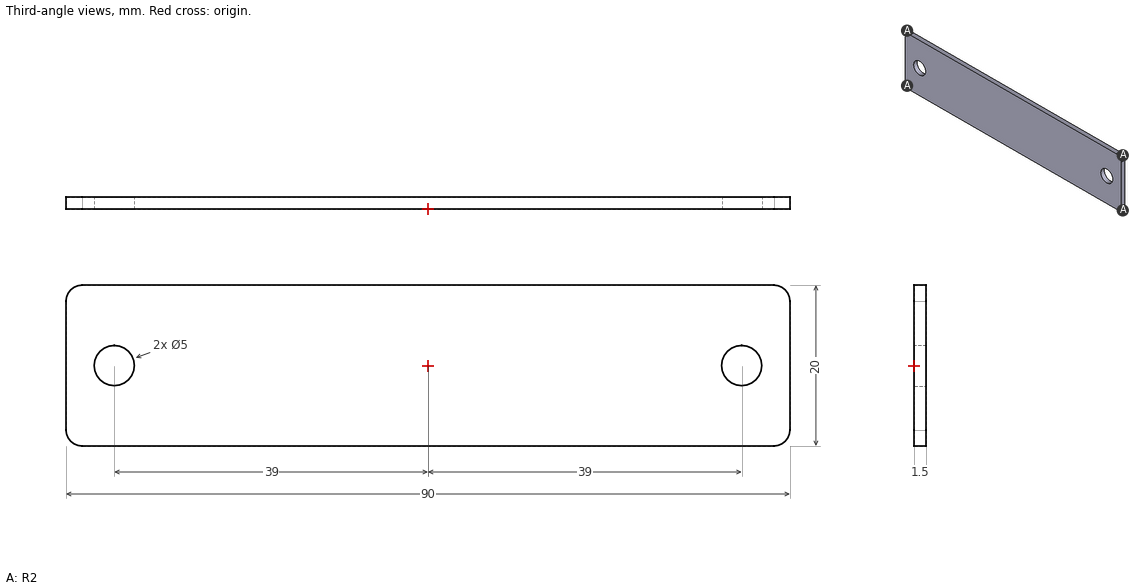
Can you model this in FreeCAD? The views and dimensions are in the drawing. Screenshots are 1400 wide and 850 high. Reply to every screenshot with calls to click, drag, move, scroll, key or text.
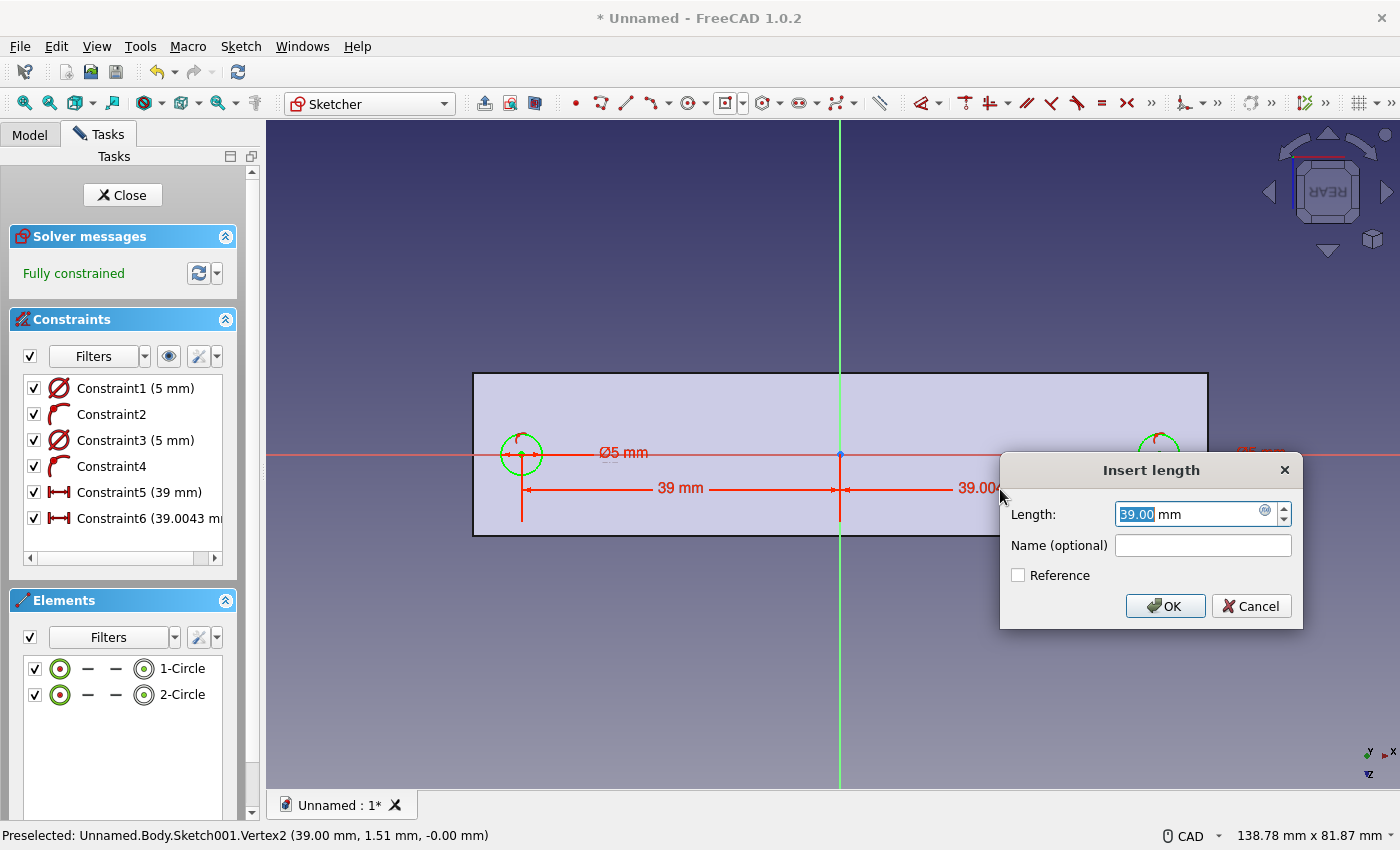
text(39)
key(Return)
key(Escape)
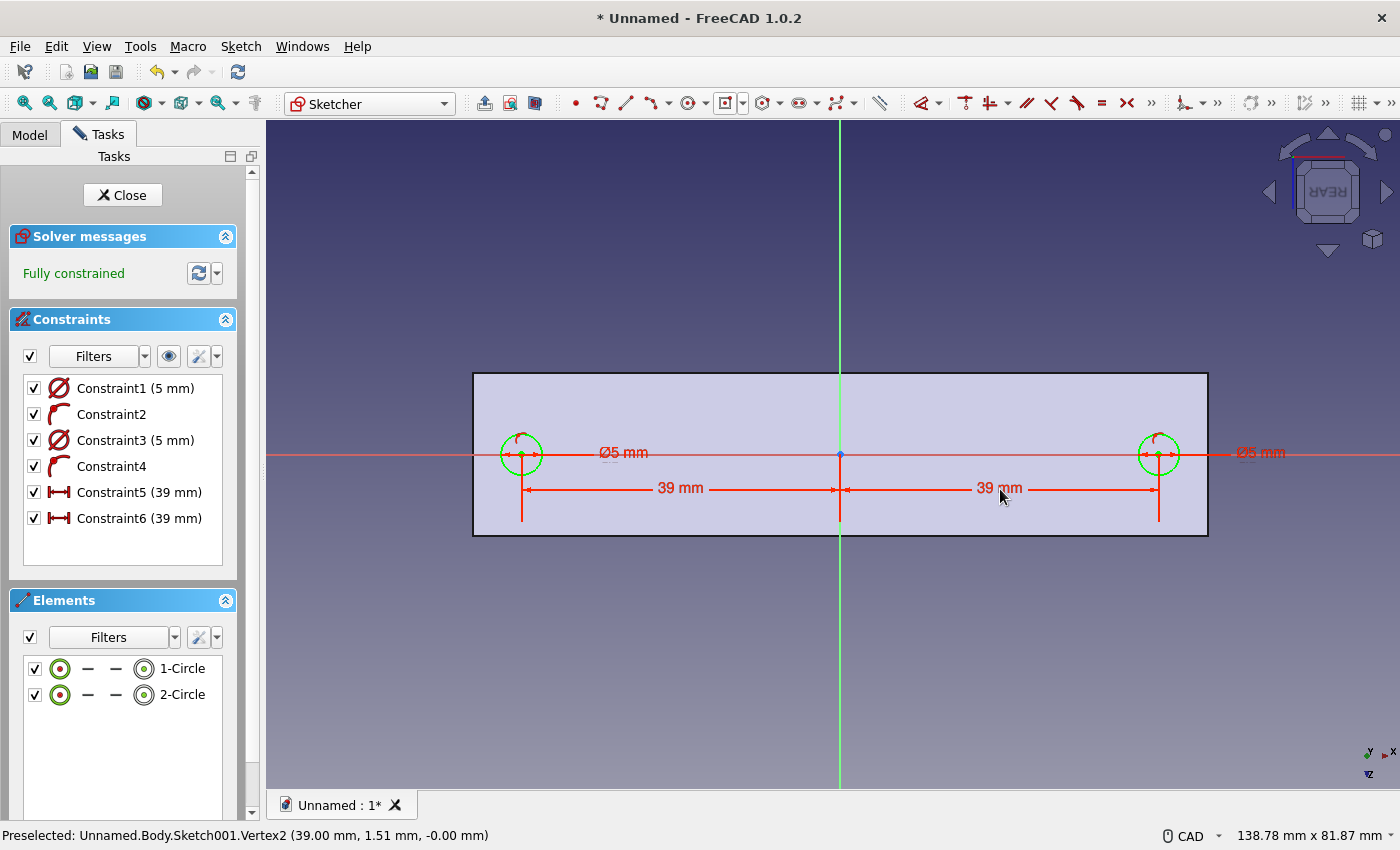
click(123, 195)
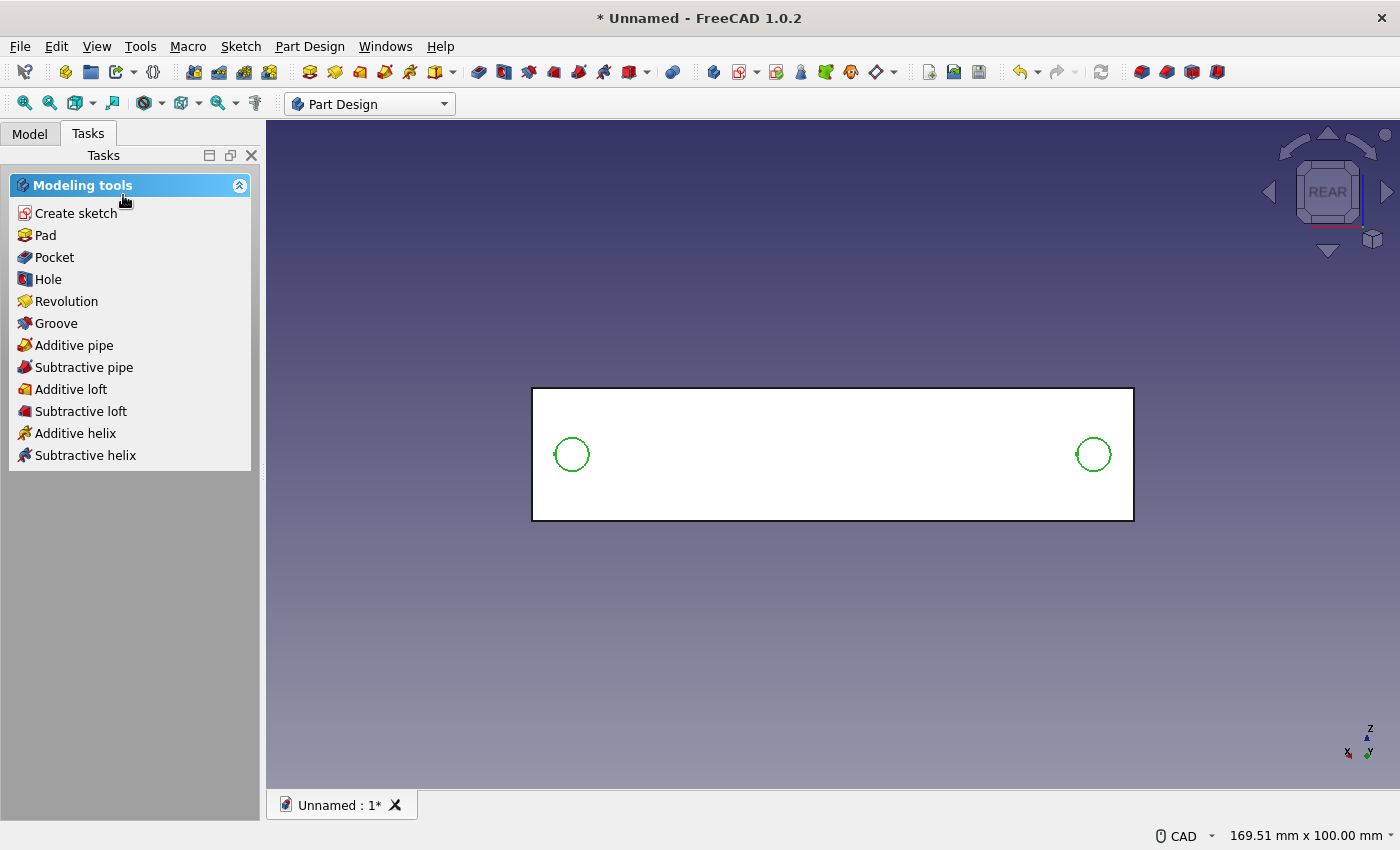
click(479, 72)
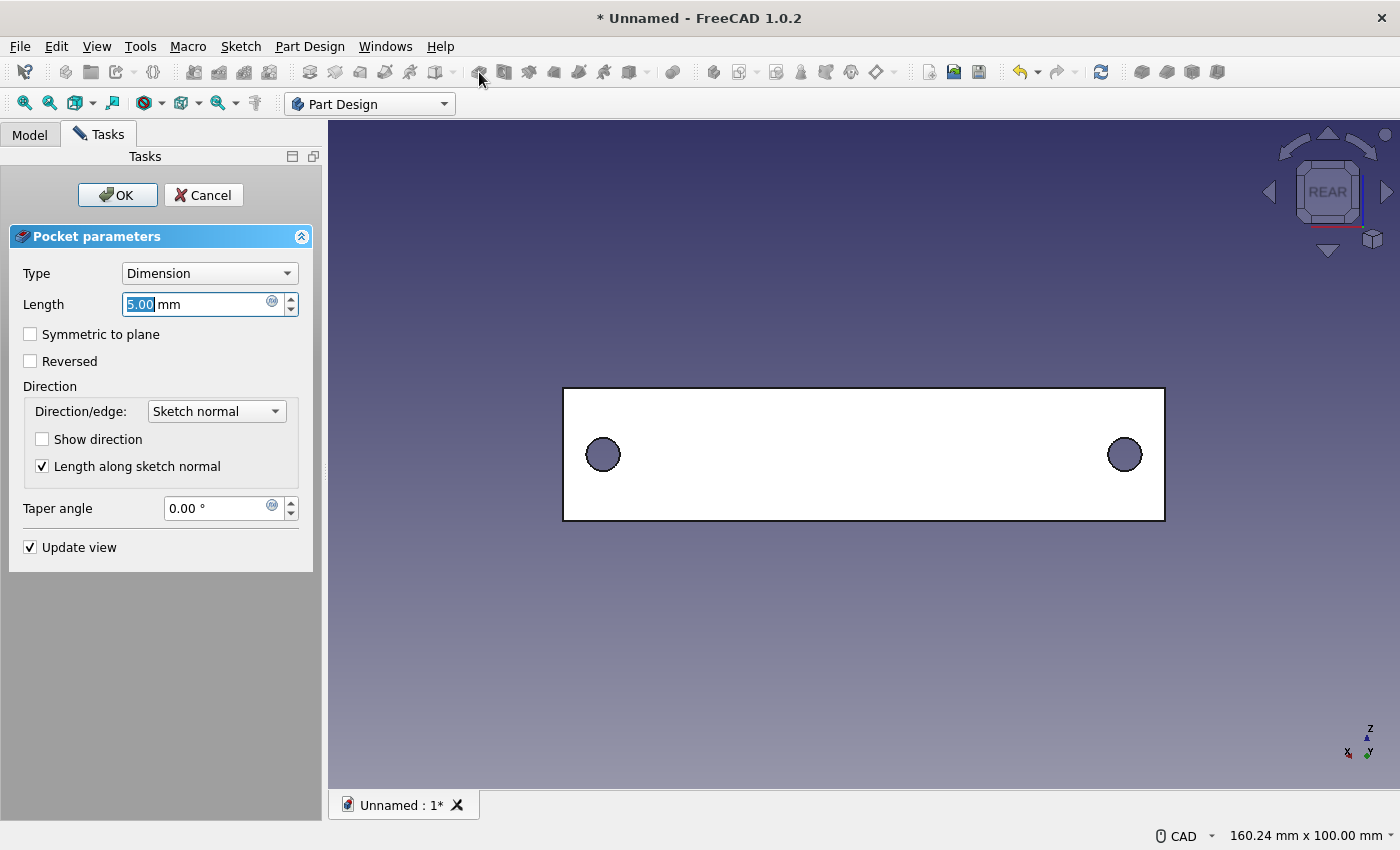
click(210, 274)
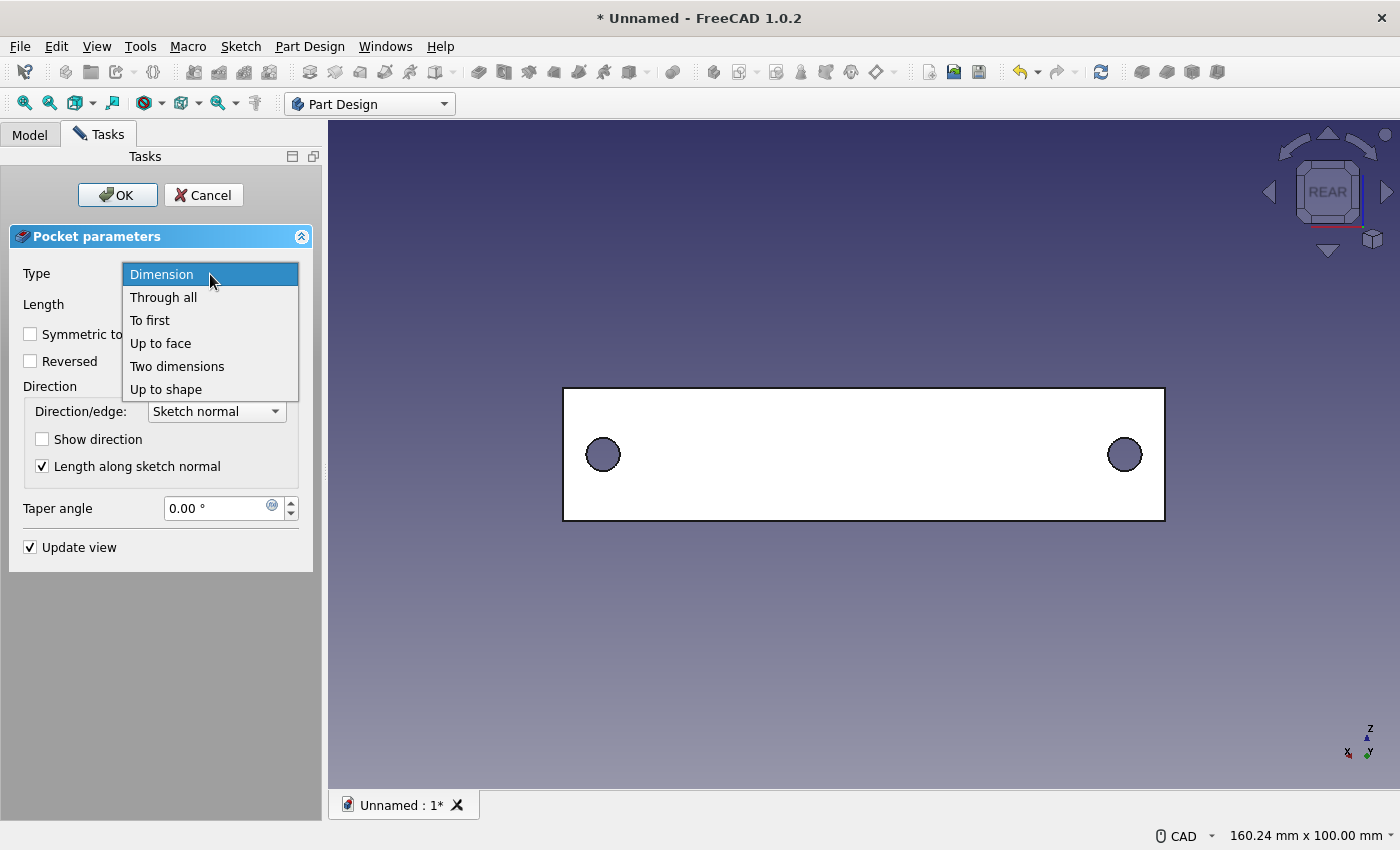
click(208, 298)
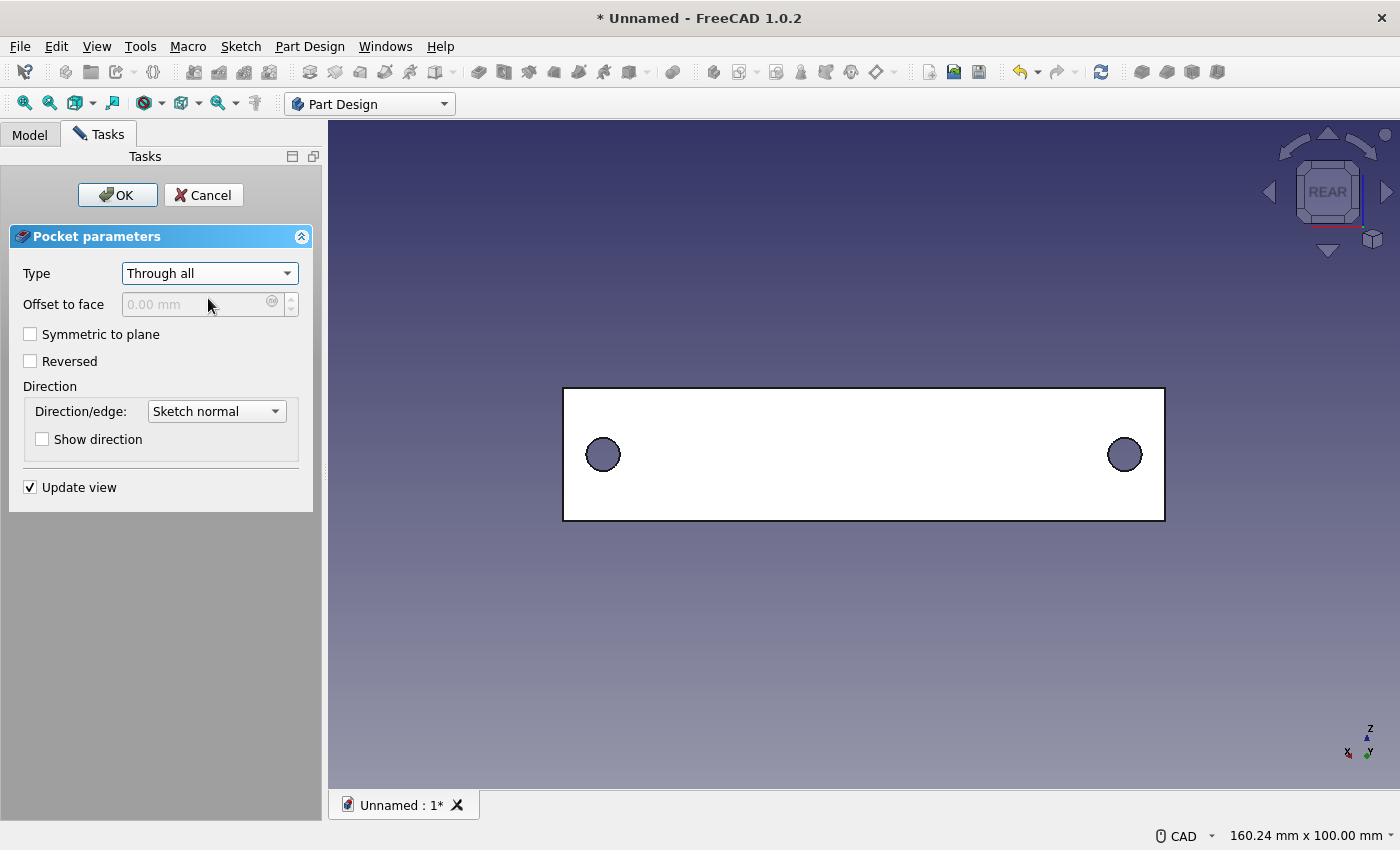
click(118, 195)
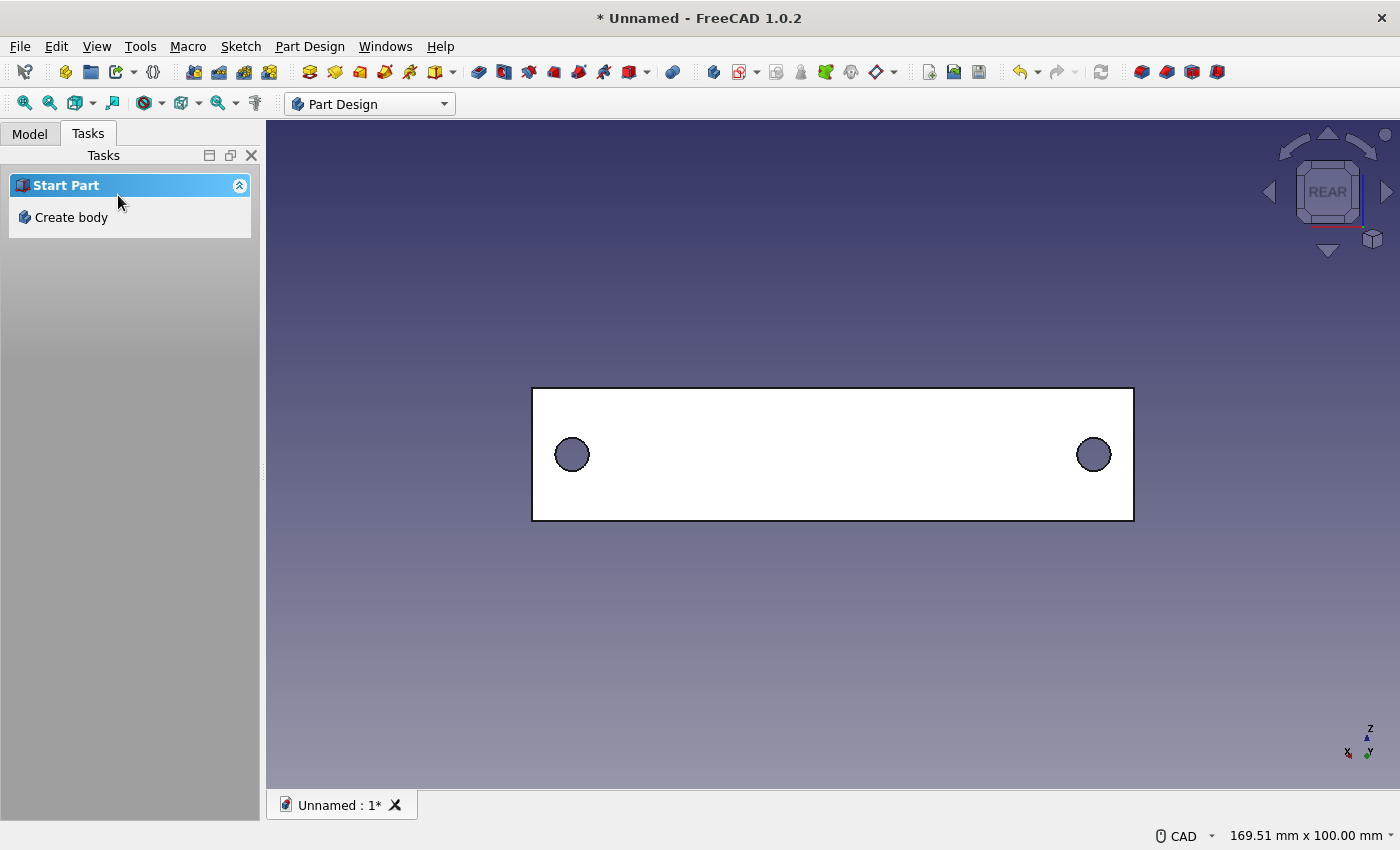
scroll(532, 387, up, 7)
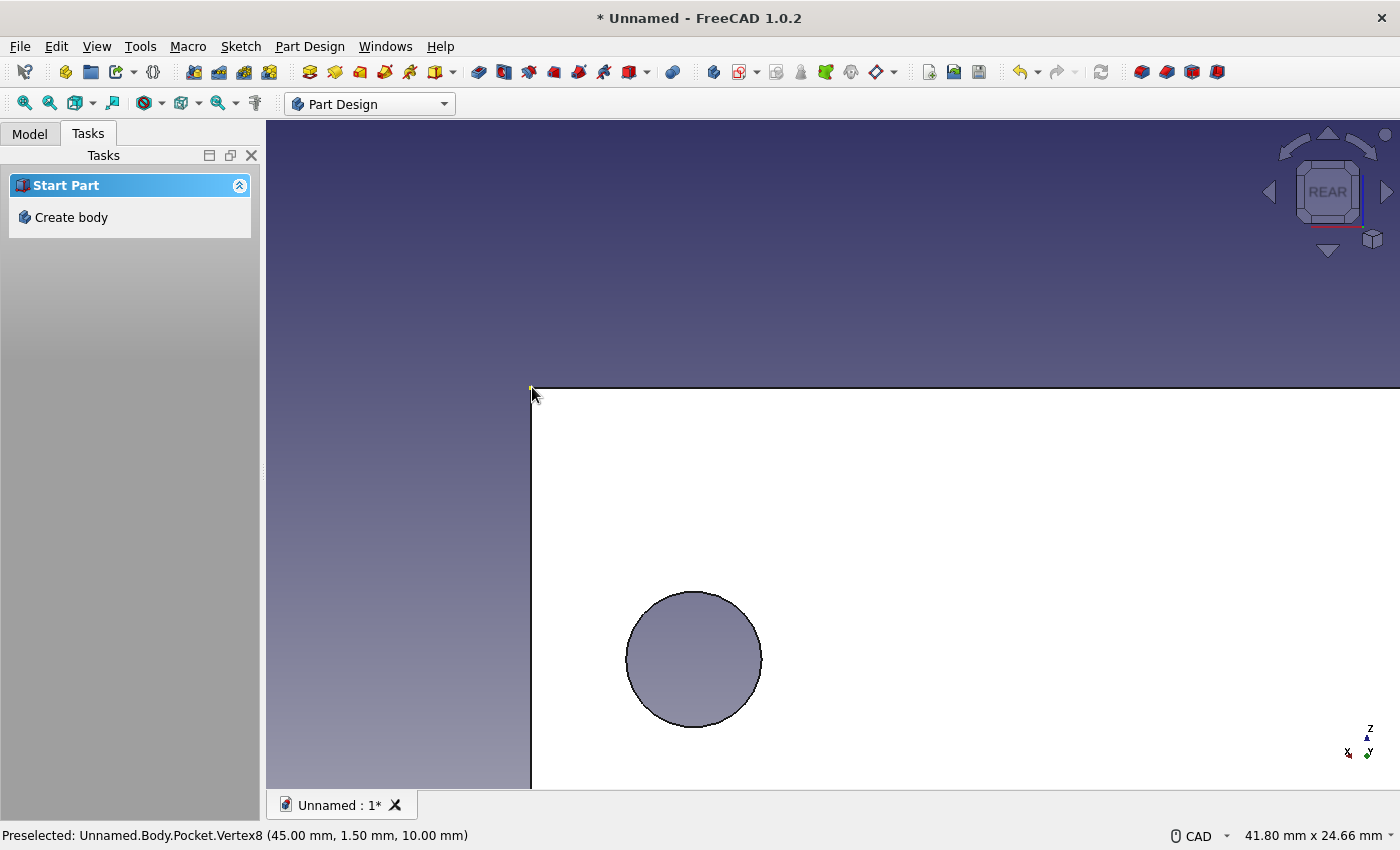
click(25, 104)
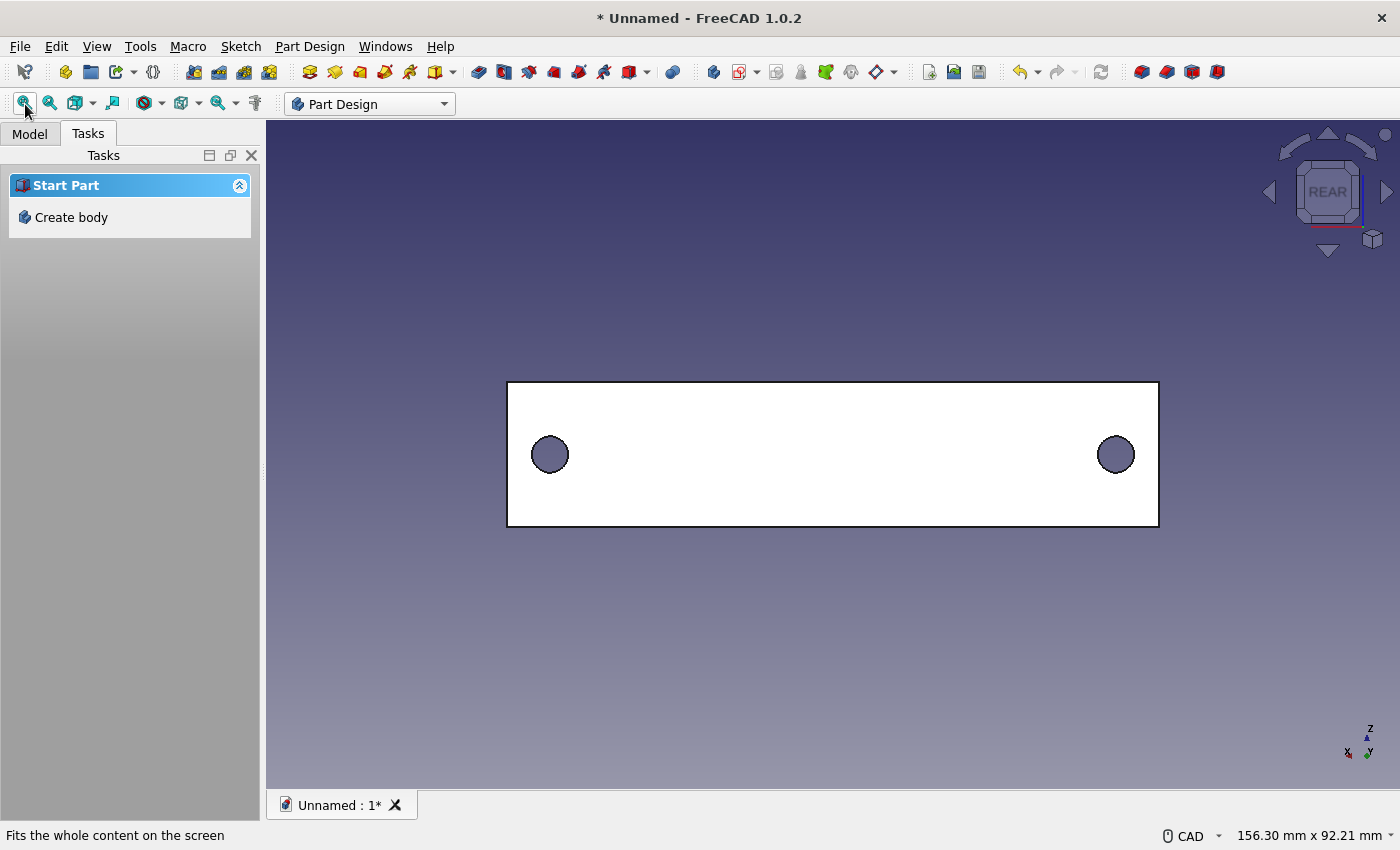
key(0)